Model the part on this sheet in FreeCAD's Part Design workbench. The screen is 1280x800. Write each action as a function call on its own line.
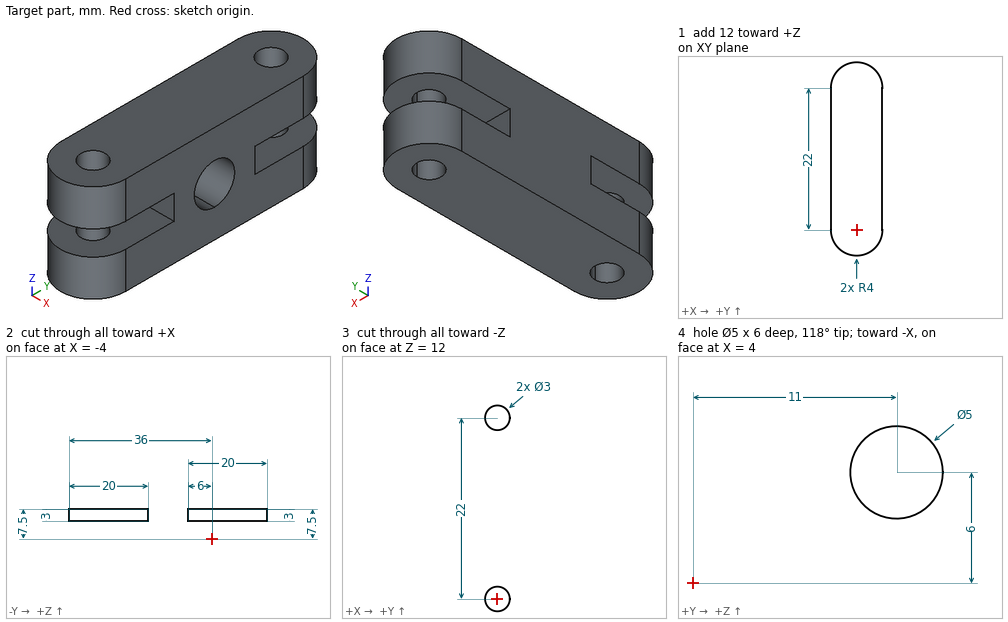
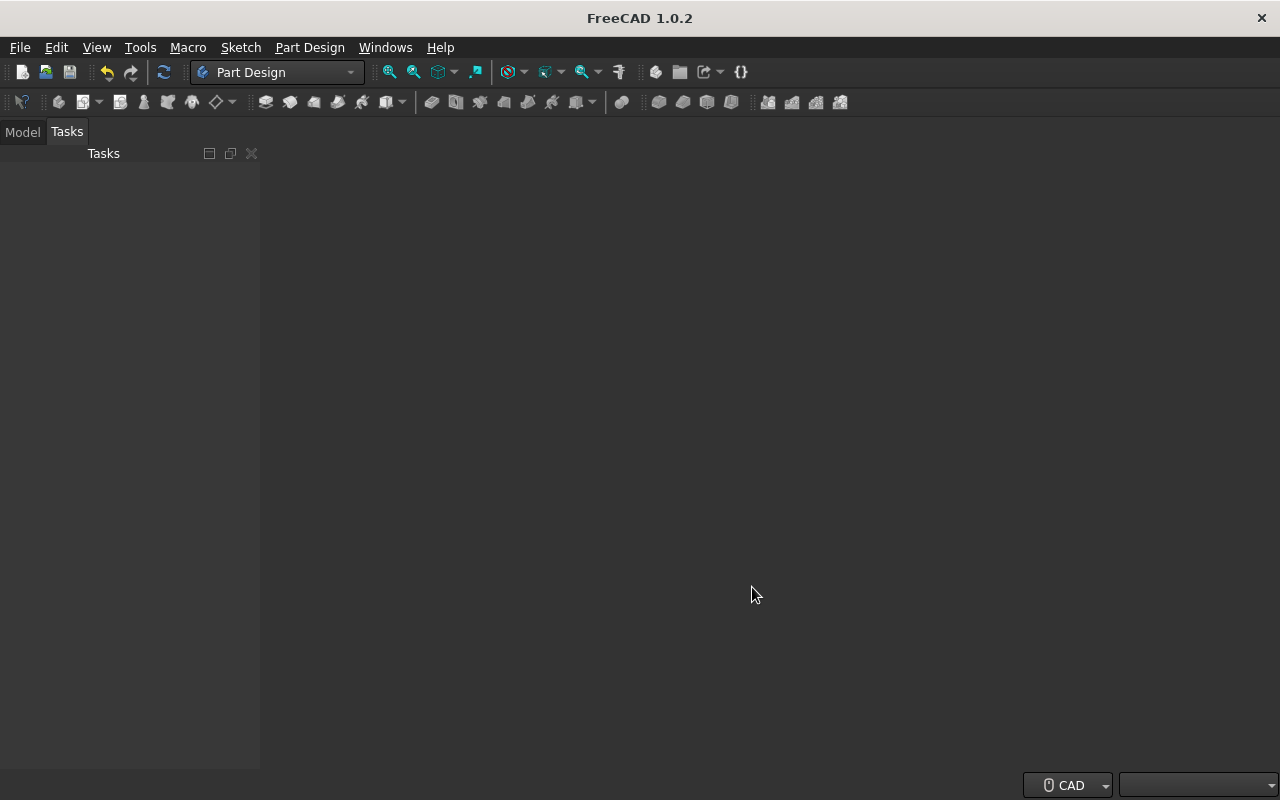
key(ctrl+n)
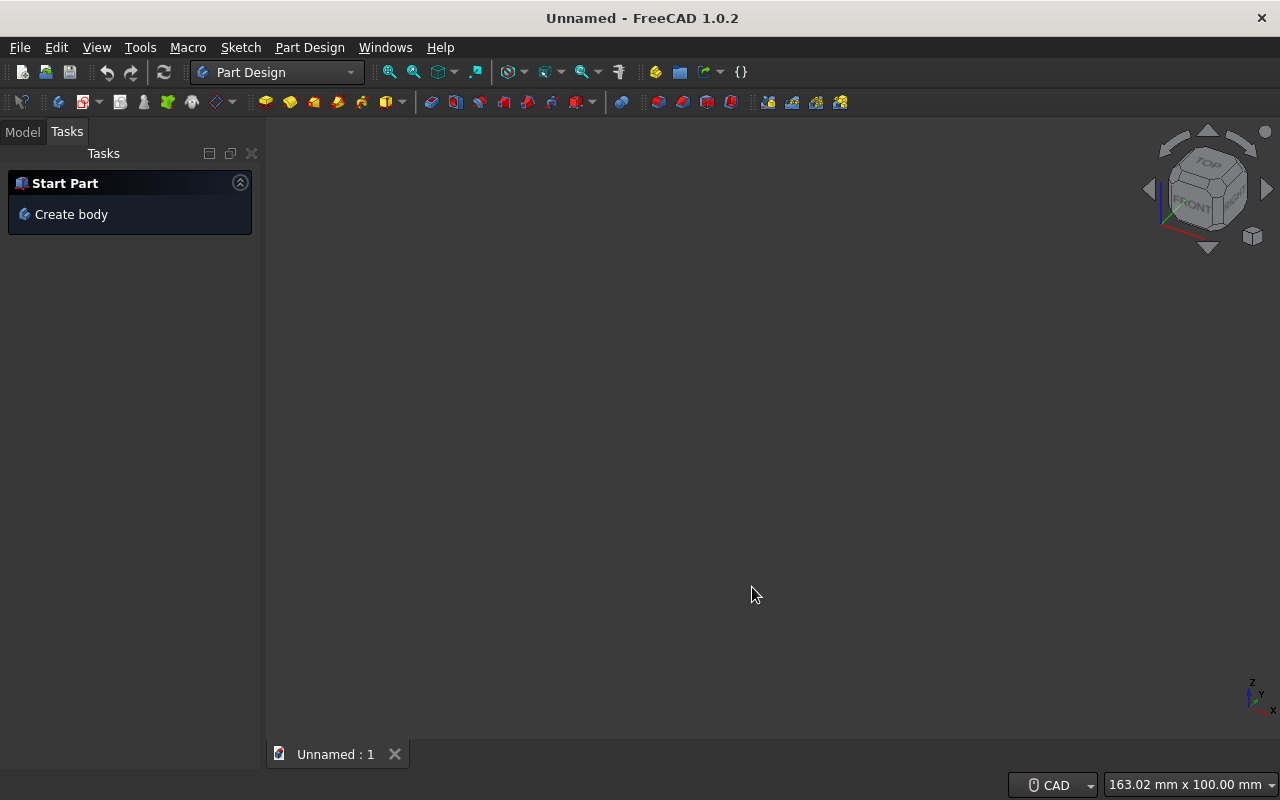
click(84, 102)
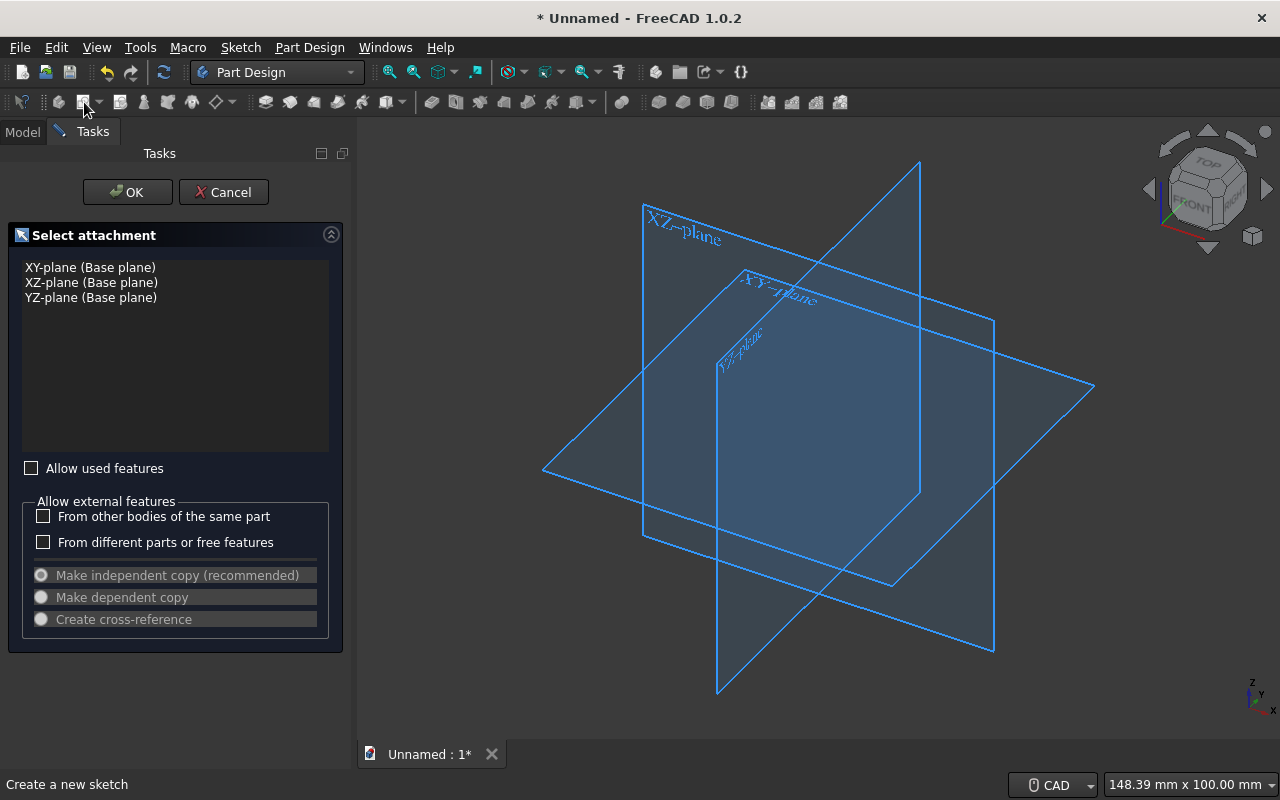
click(82, 268)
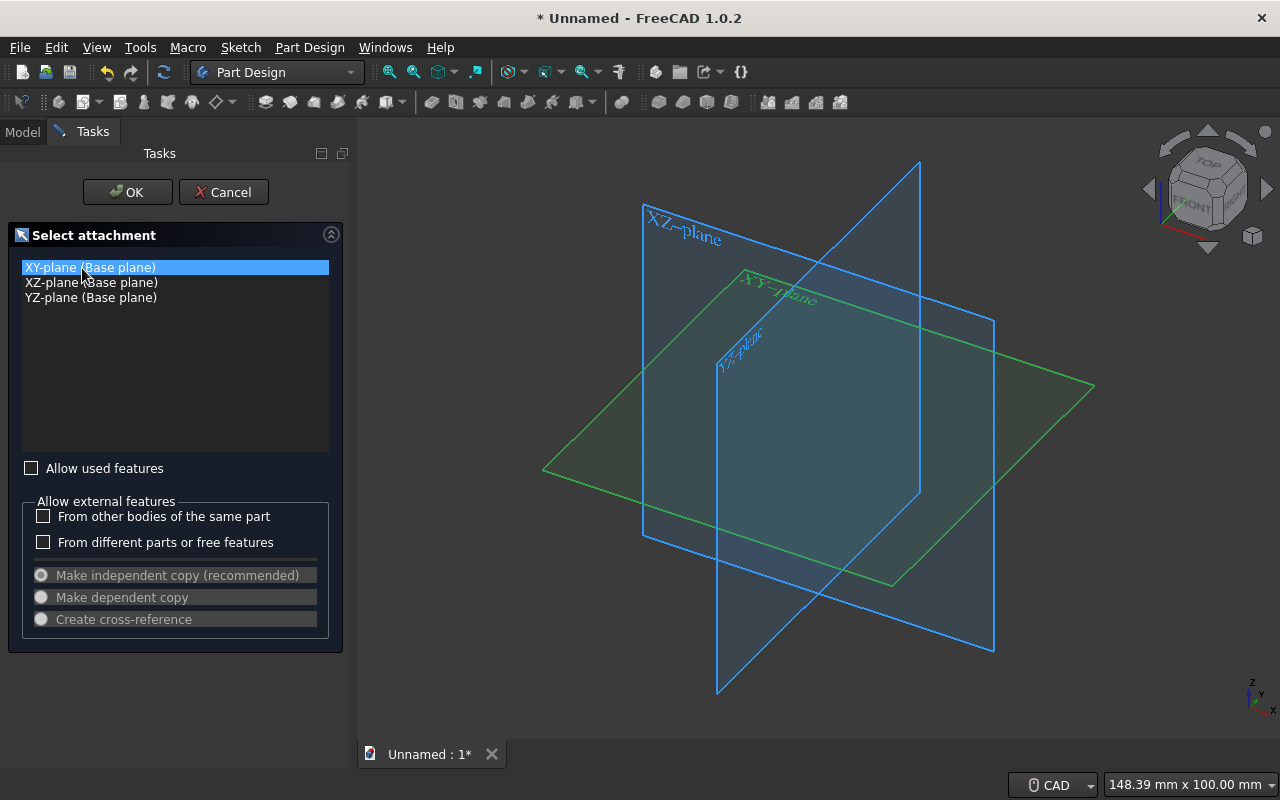
click(128, 192)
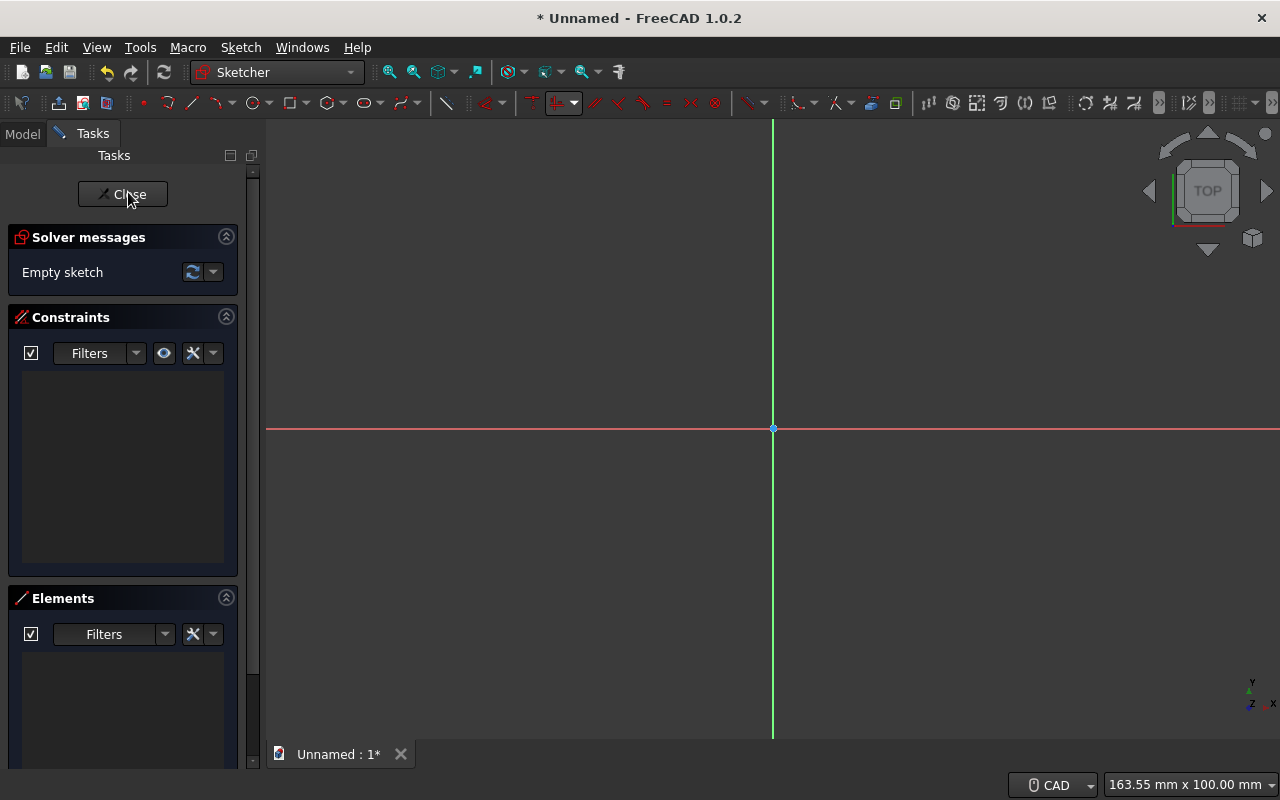
scroll(829, 305, up, 4)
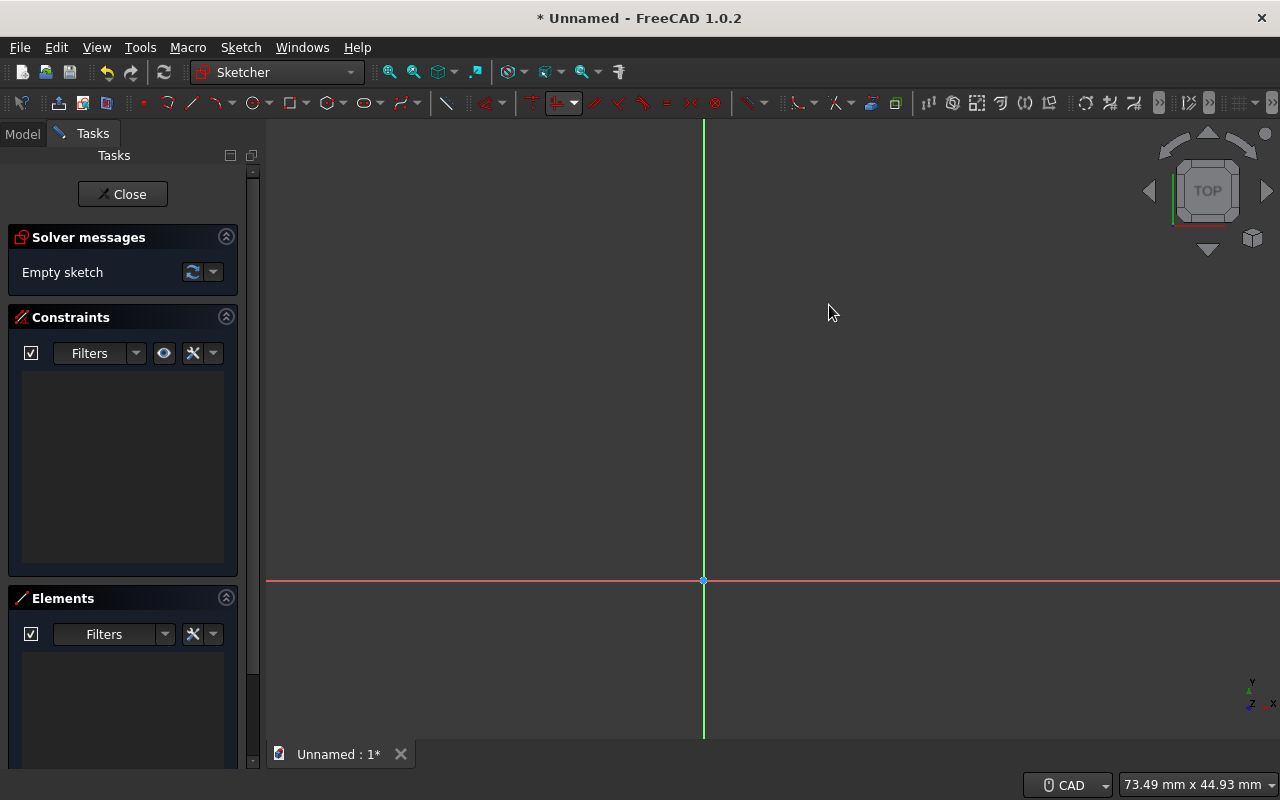
key(g)
key(s)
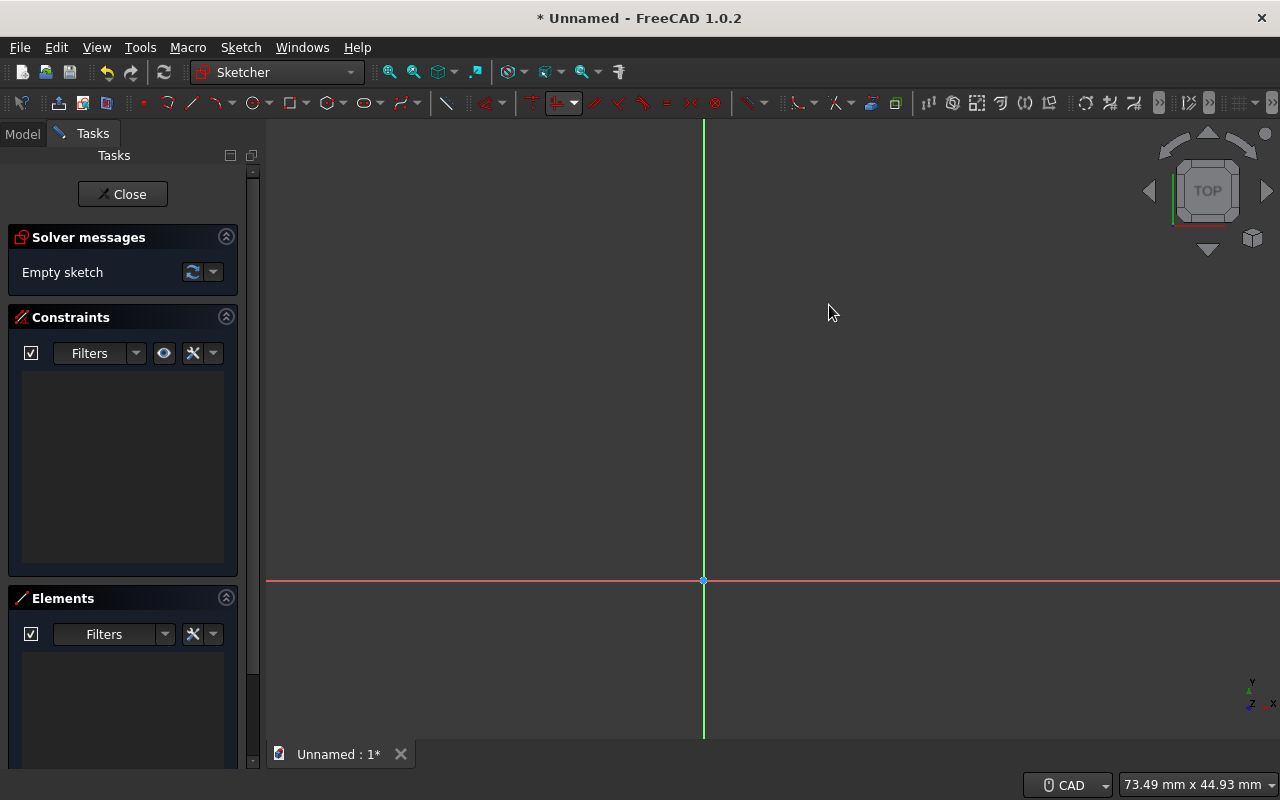
click(704, 581)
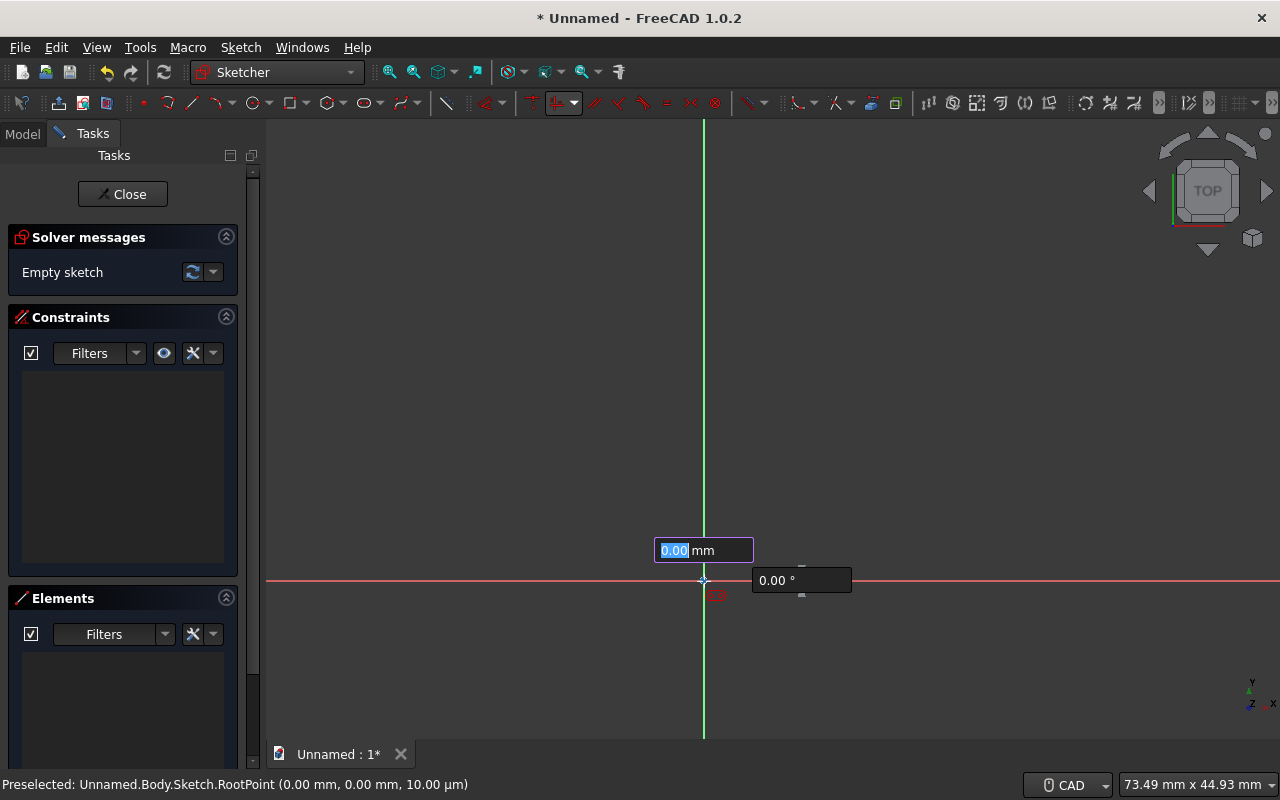
click(713, 277)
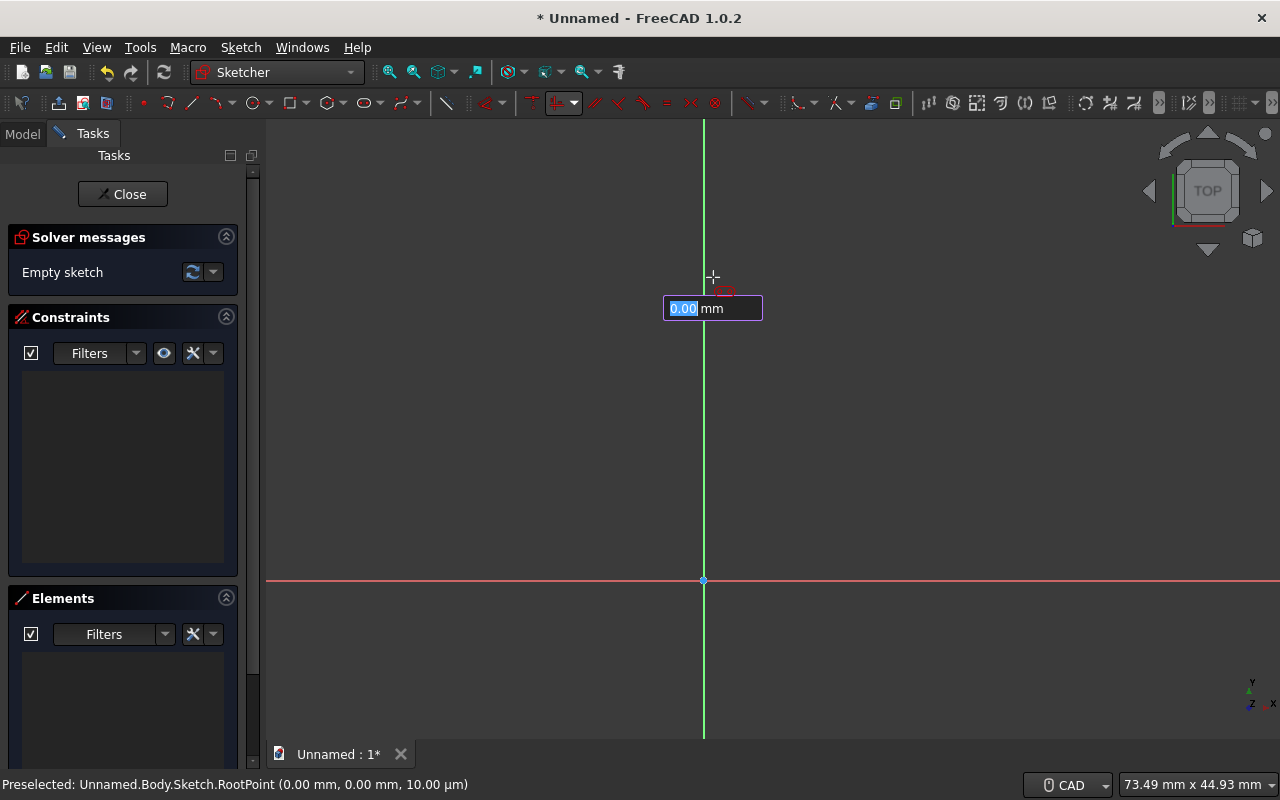
click(648, 429)
key(Escape)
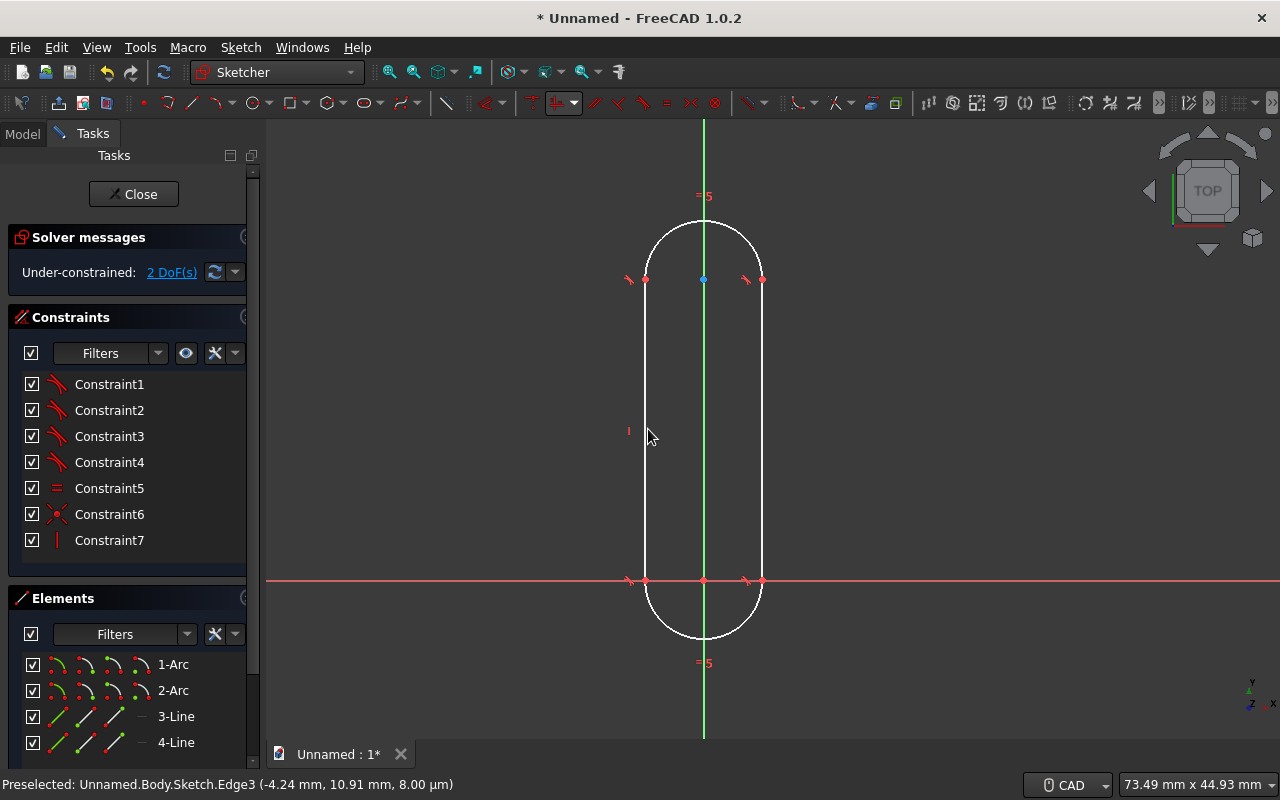
key(d)